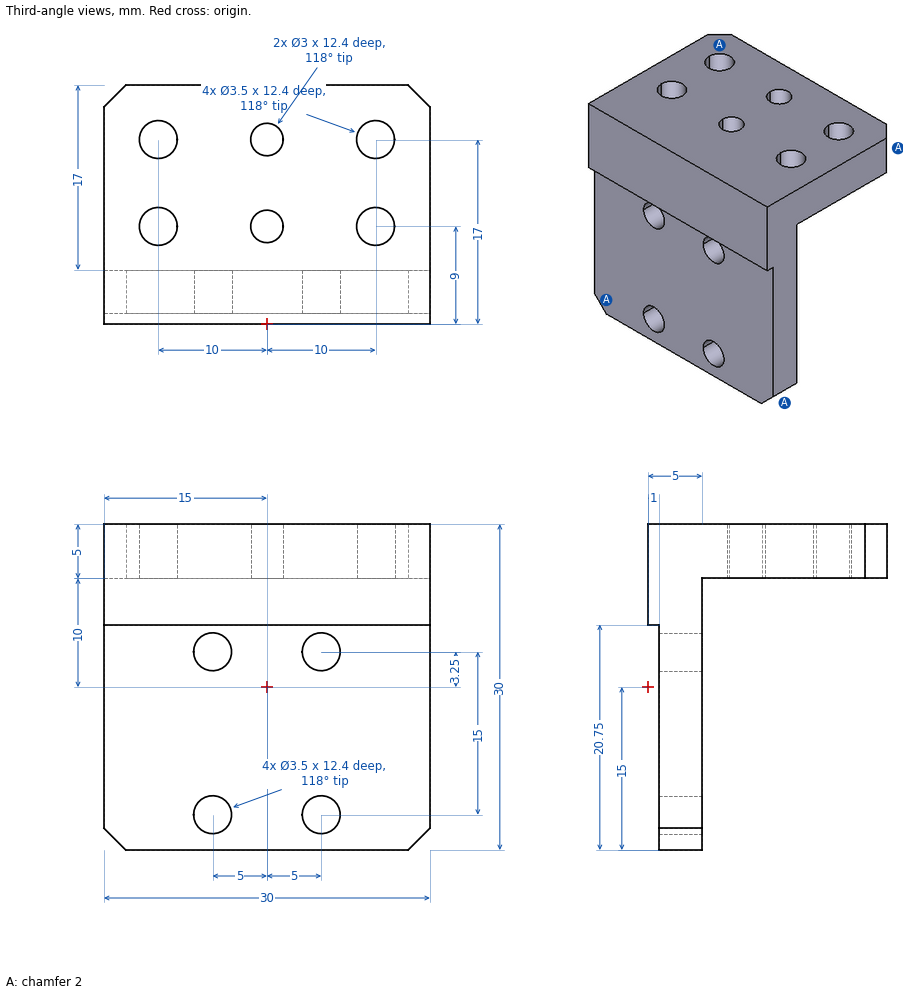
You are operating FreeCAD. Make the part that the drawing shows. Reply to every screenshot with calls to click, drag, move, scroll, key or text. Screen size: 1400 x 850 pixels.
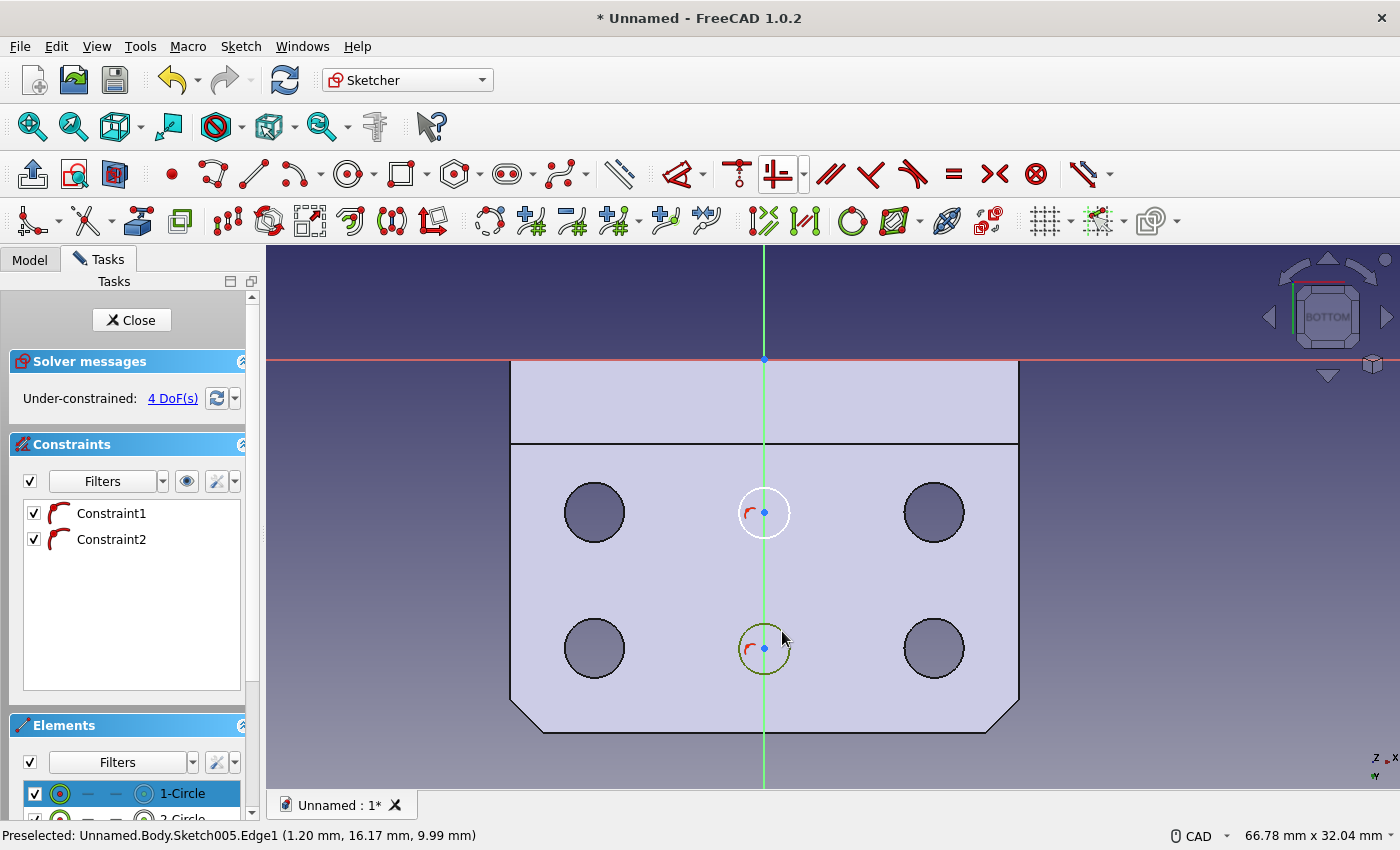
click(782, 495)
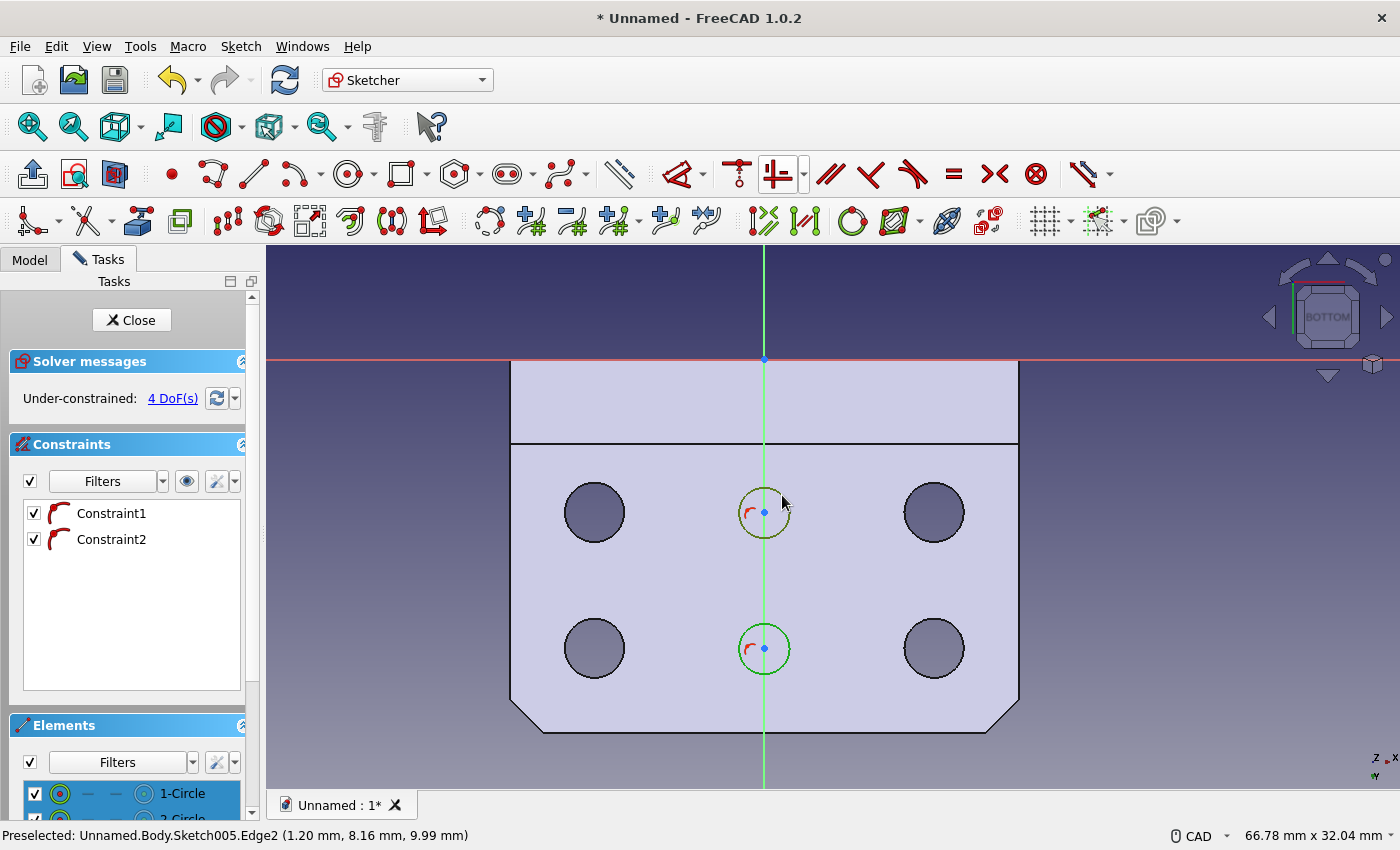
key(e)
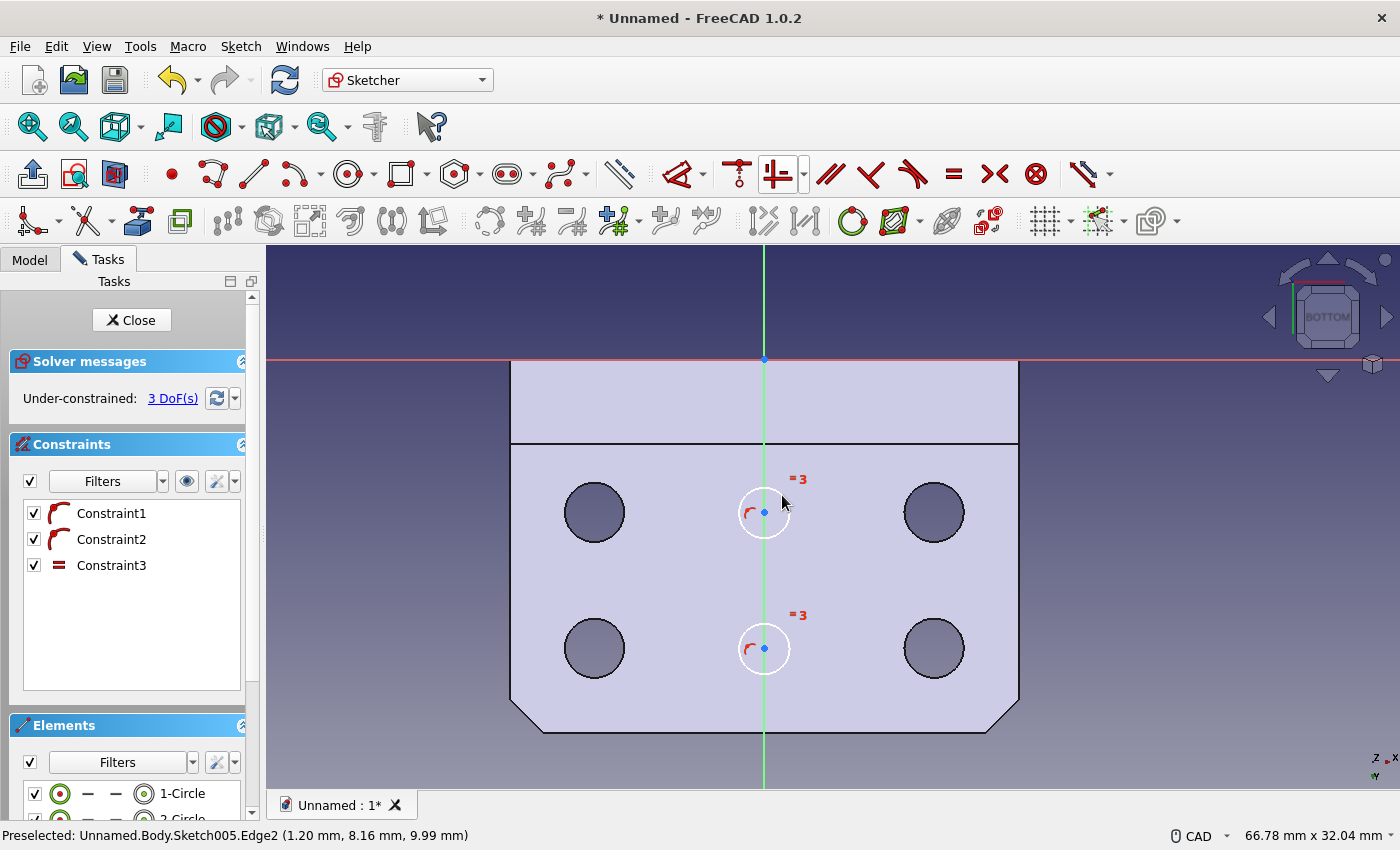
key(d)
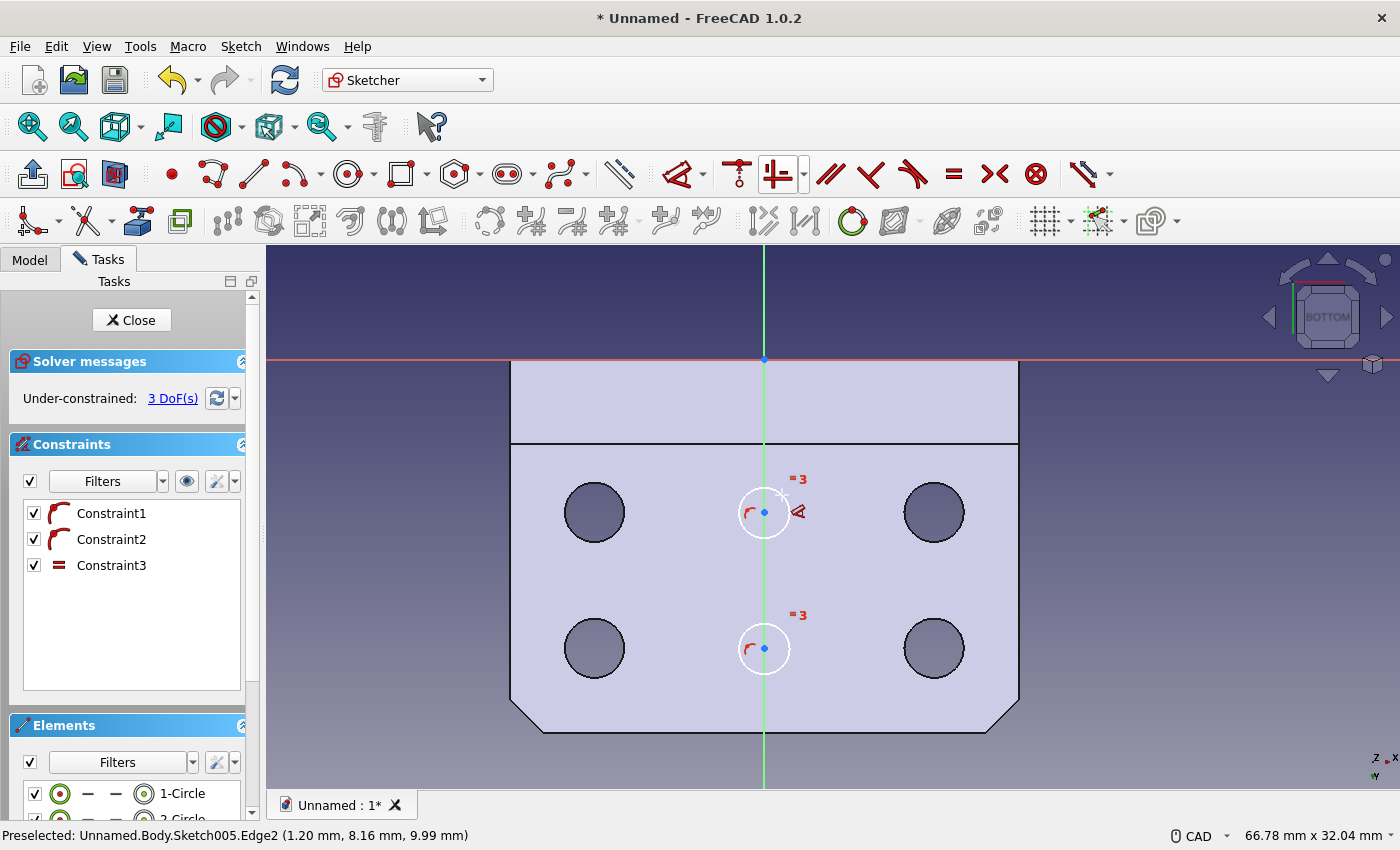
click(782, 631)
click(804, 608)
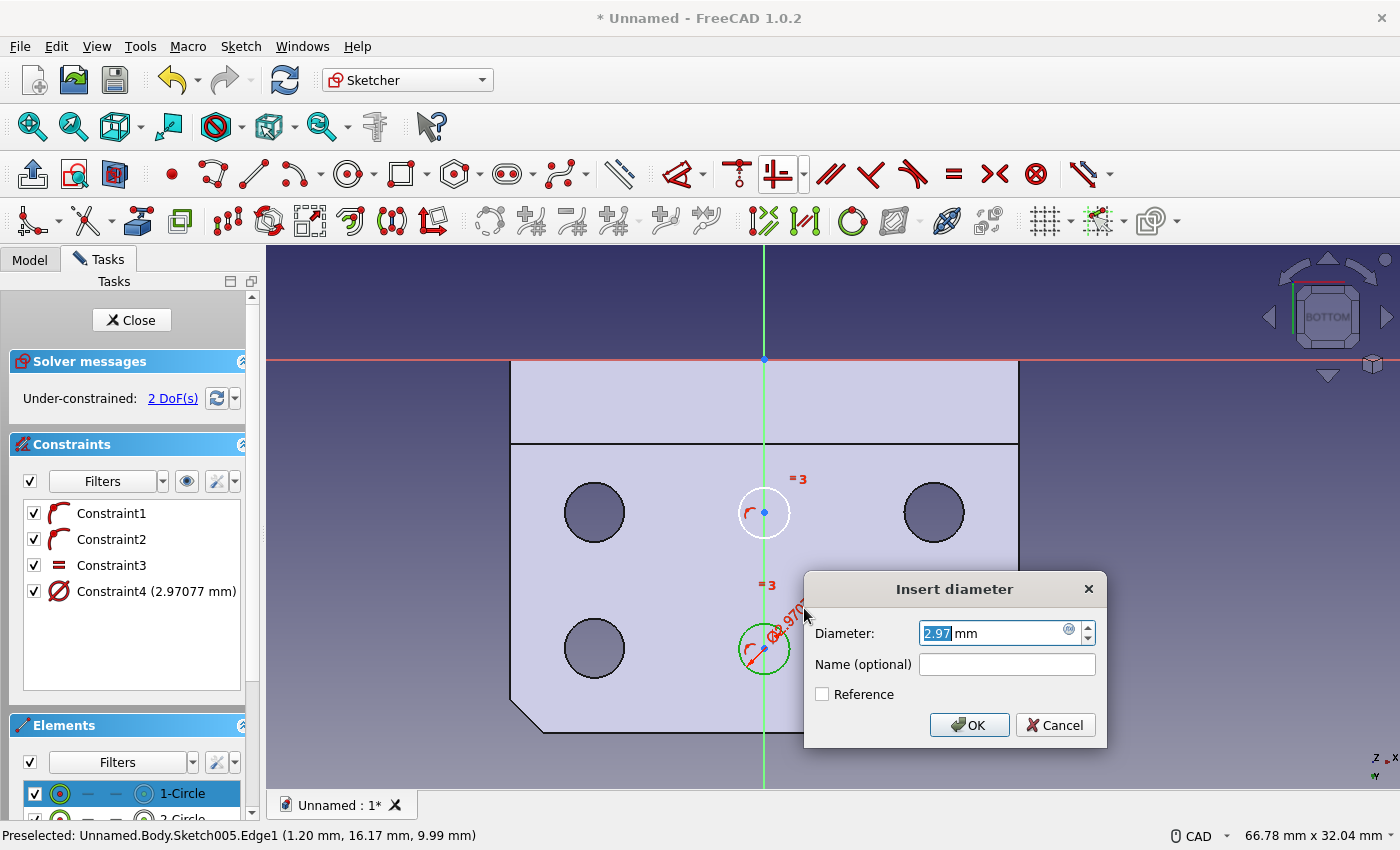
text(3)
key(Return)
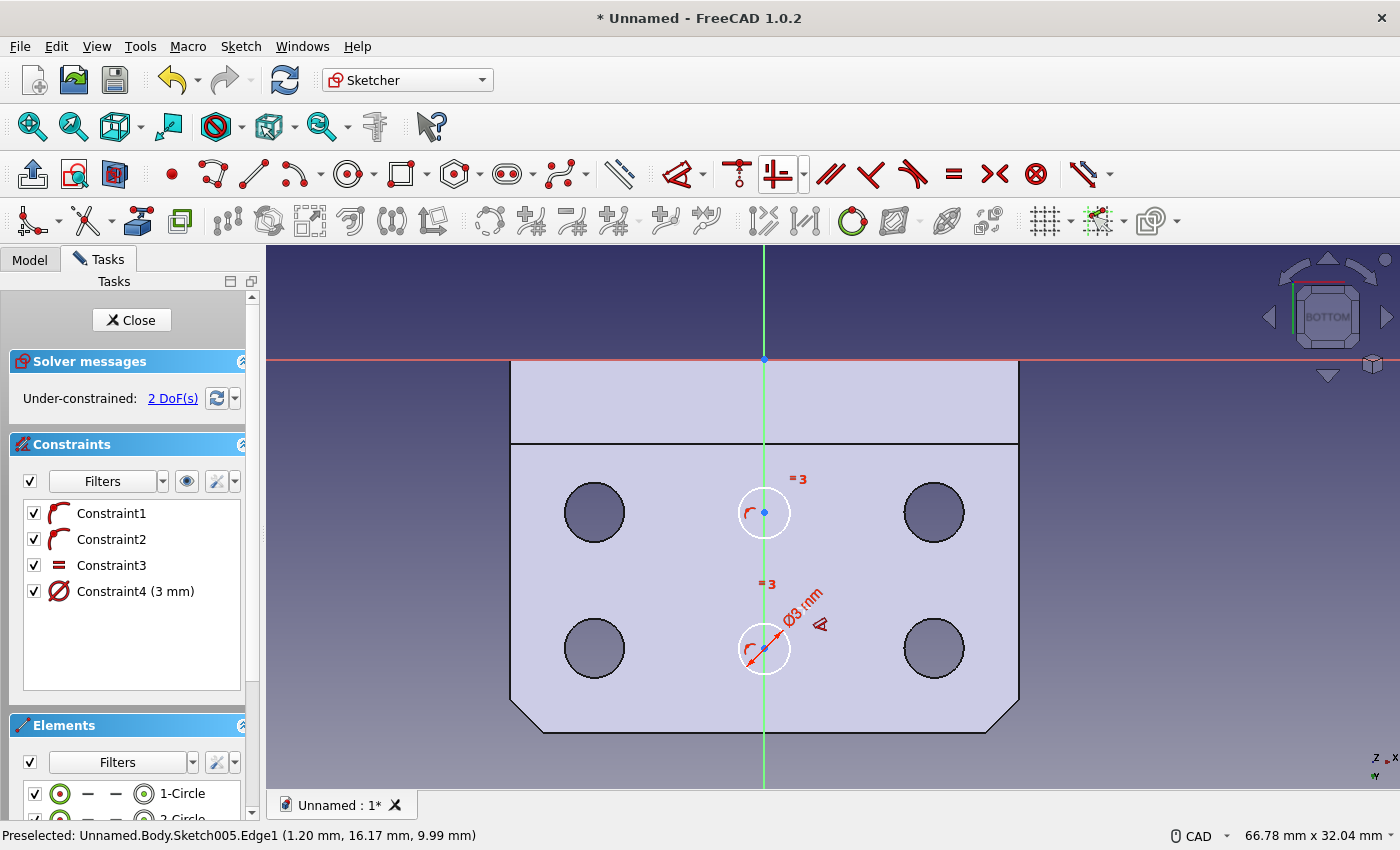
click(764, 513)
click(798, 436)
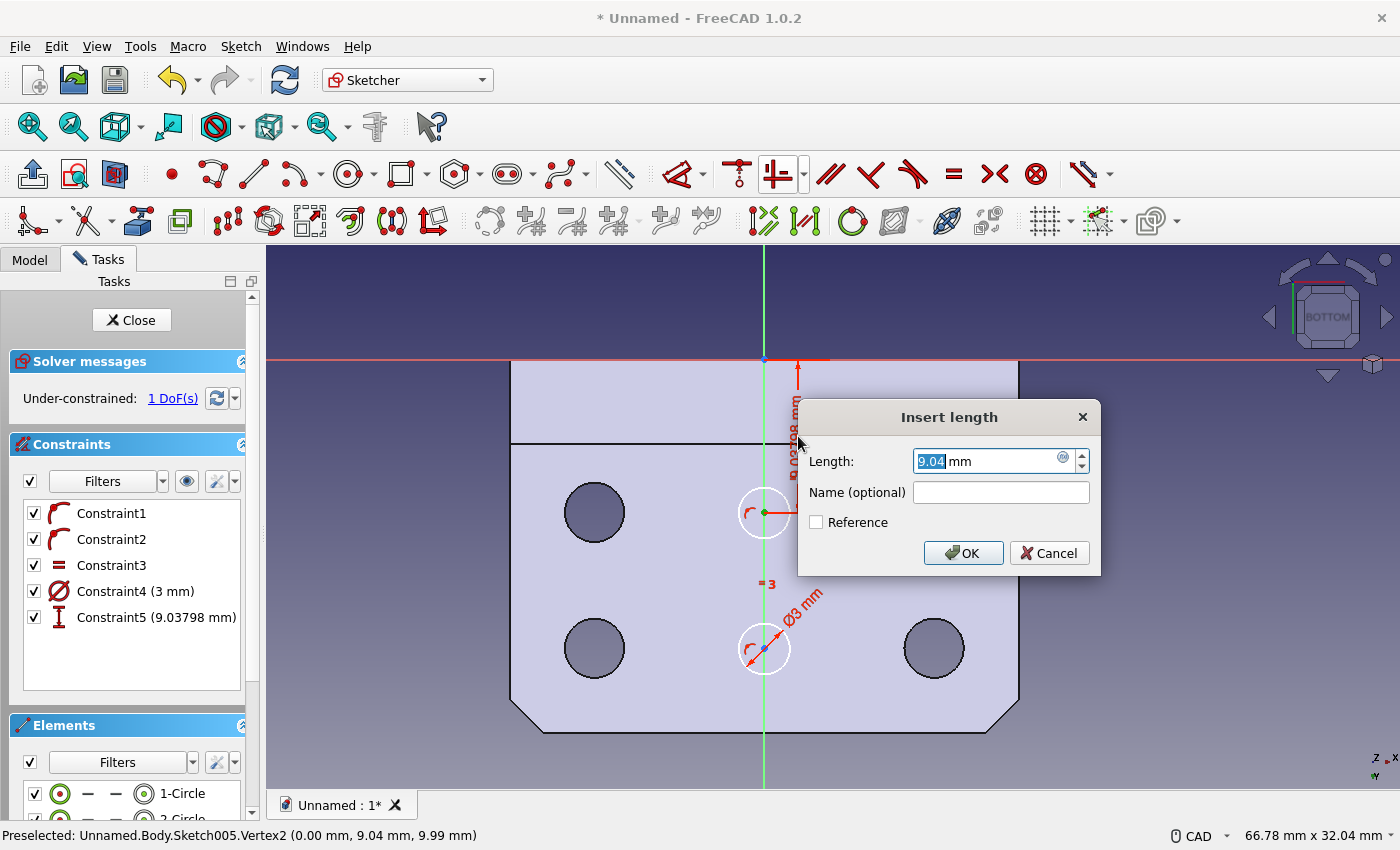
text(9)
key(Return)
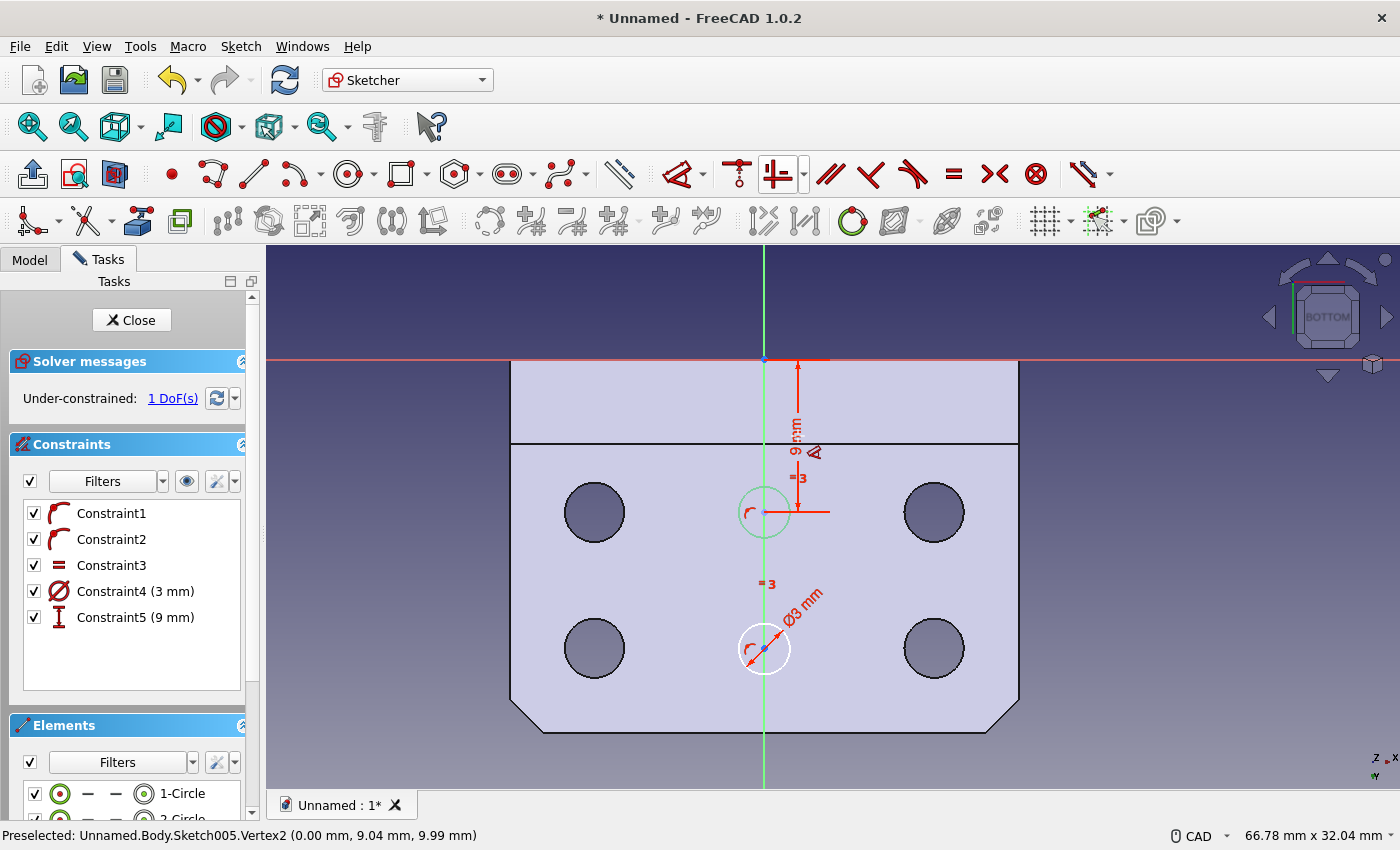
click(764, 649)
click(798, 571)